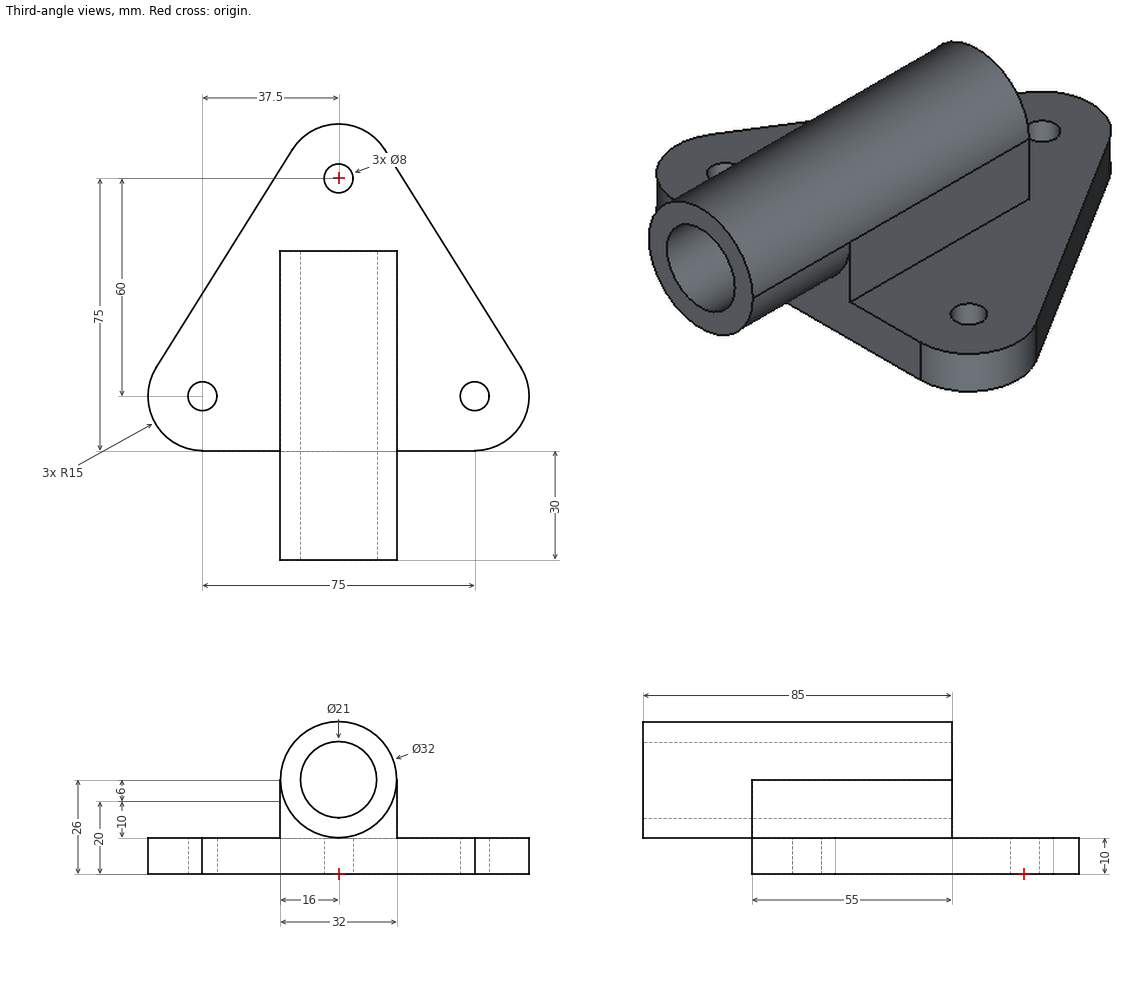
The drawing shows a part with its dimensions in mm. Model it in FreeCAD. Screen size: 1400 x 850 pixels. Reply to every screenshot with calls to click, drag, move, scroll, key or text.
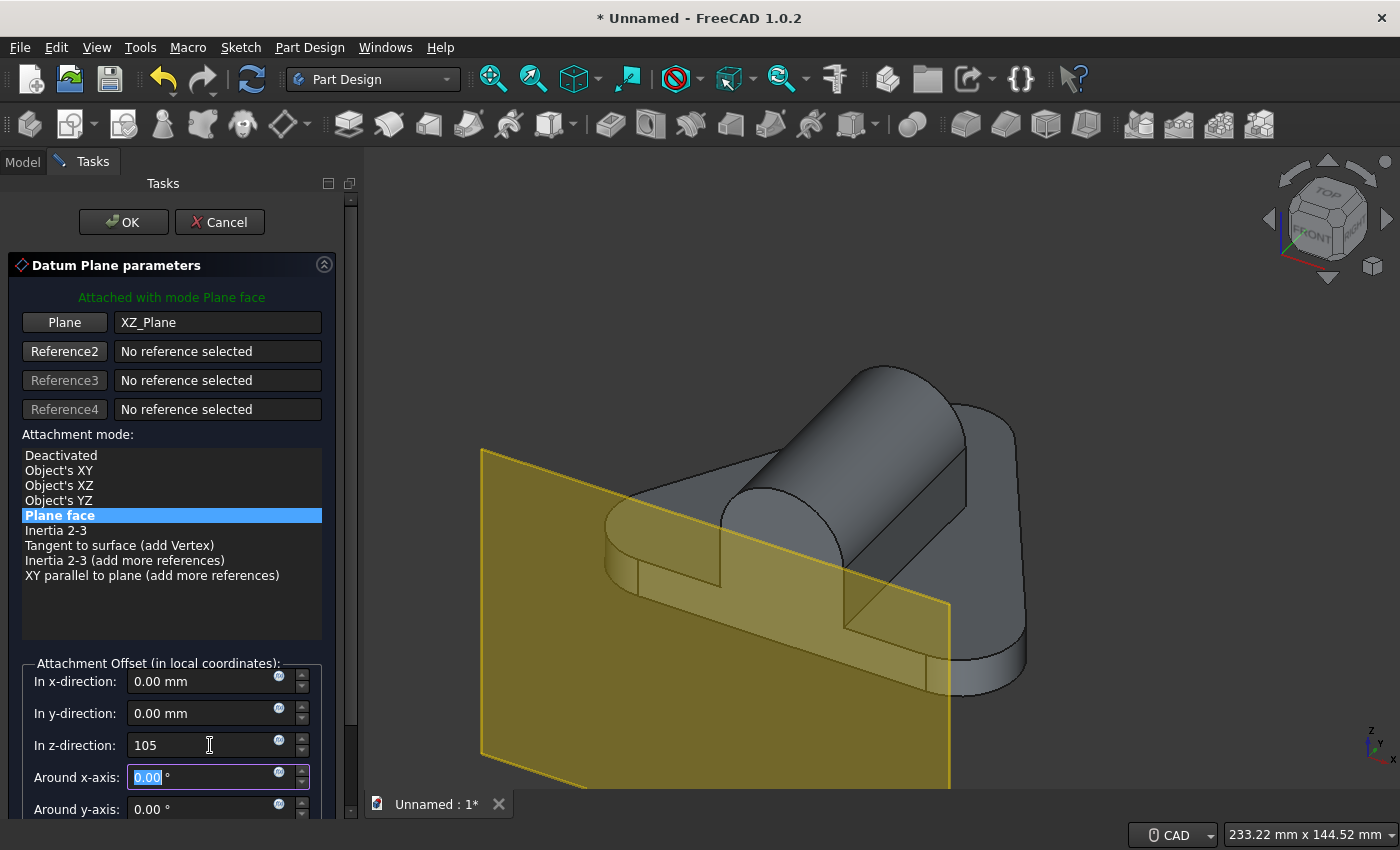
click(124, 222)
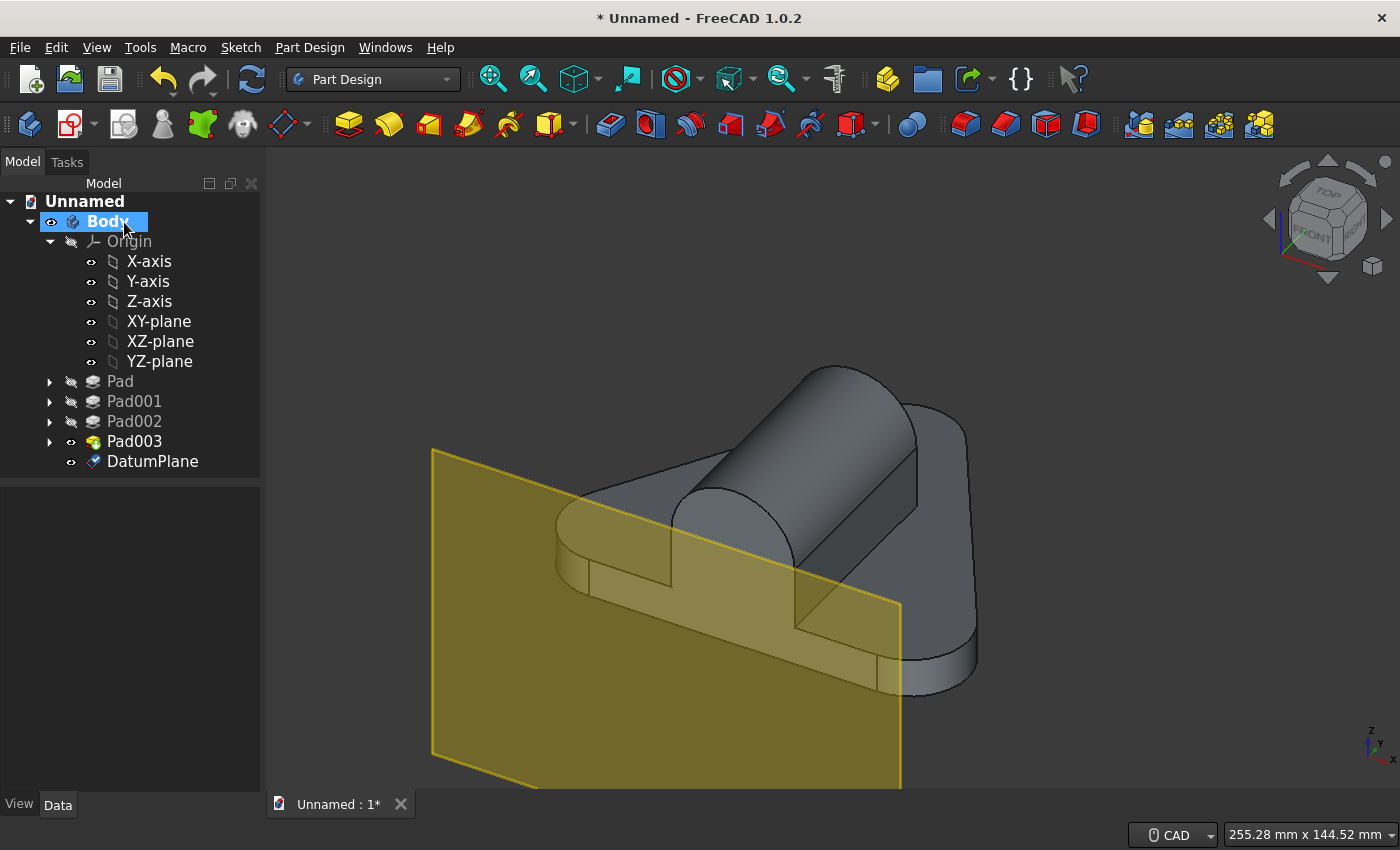
click(116, 462)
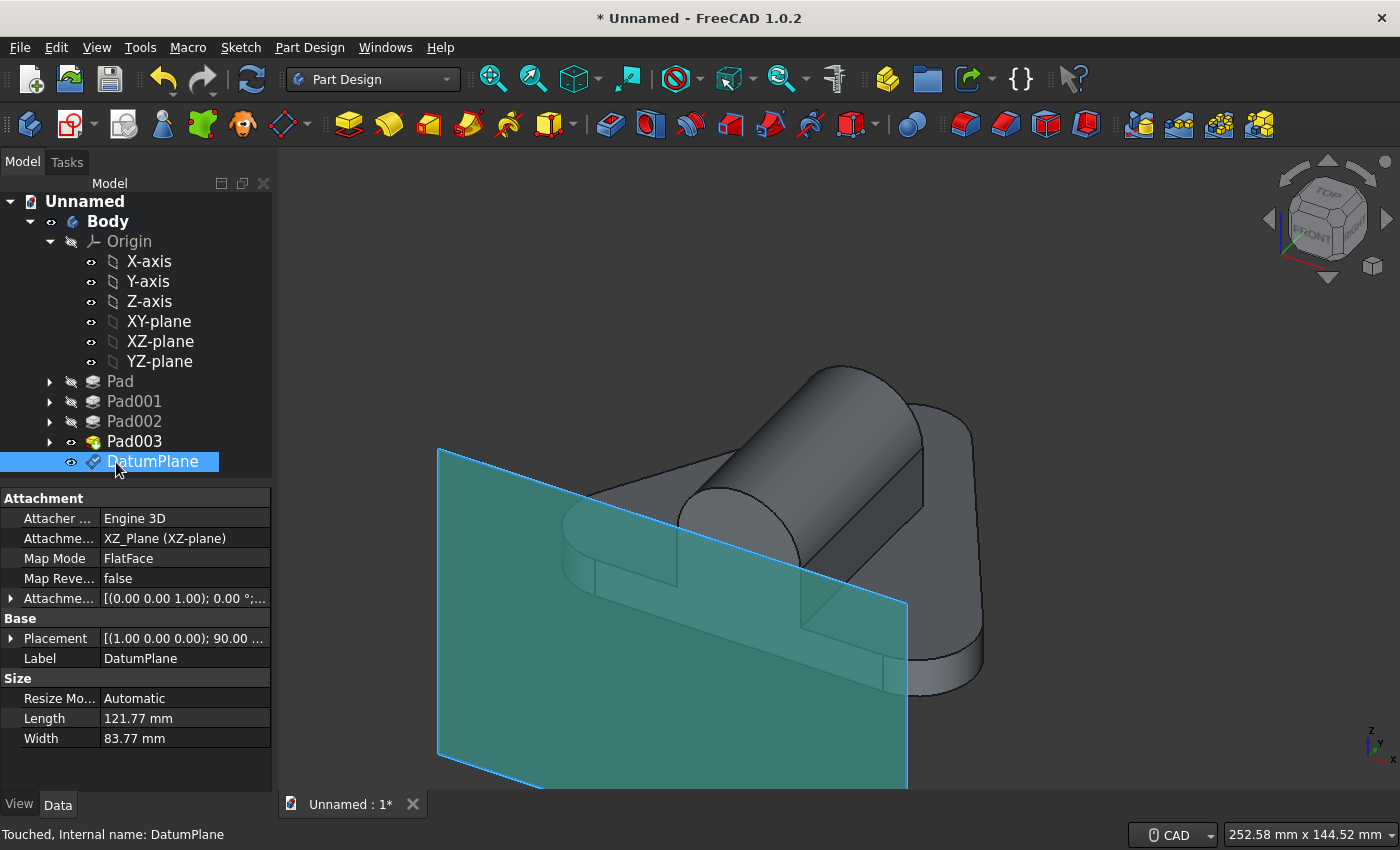
click(70, 124)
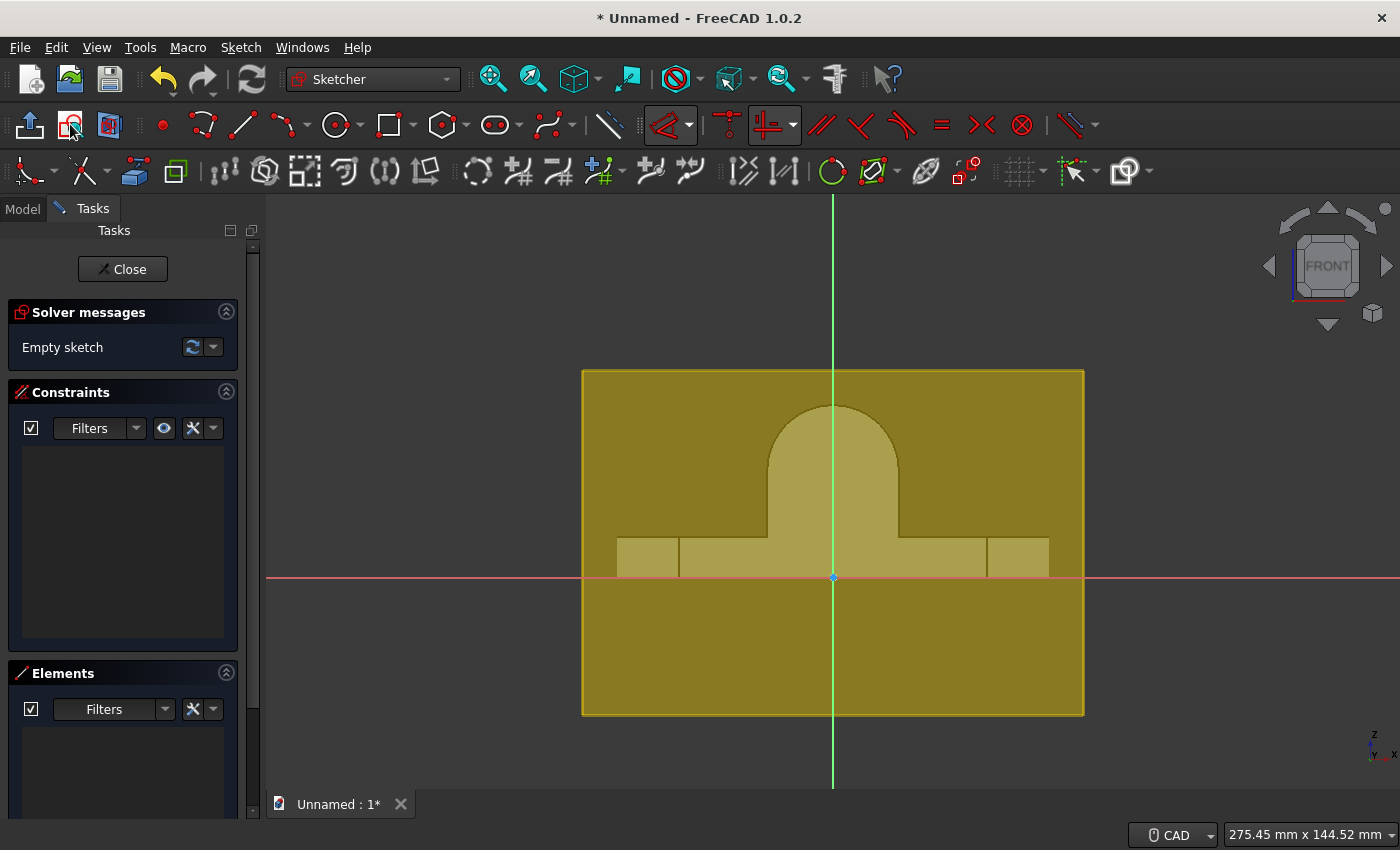
scroll(889, 491, up, 4)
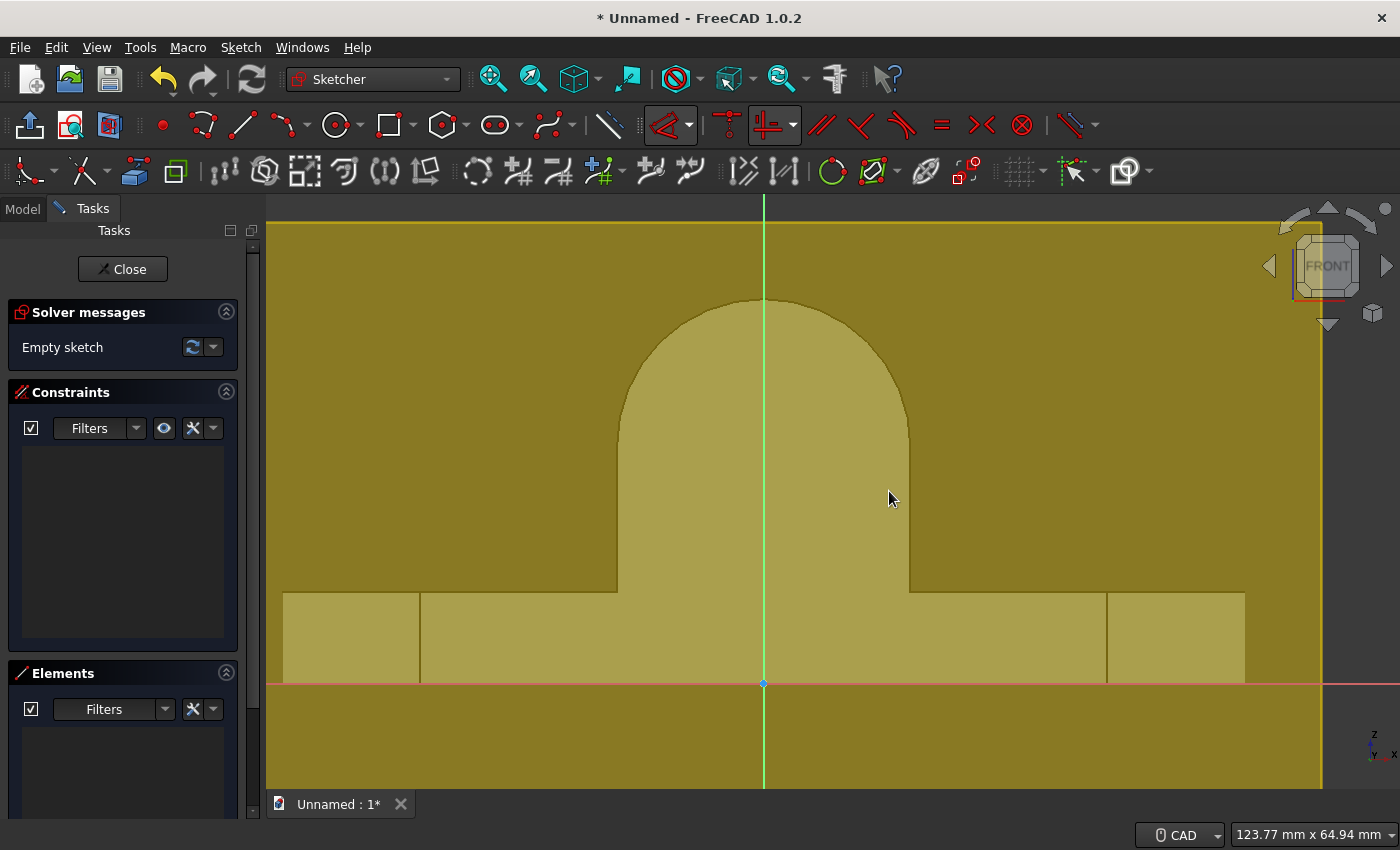
click(336, 126)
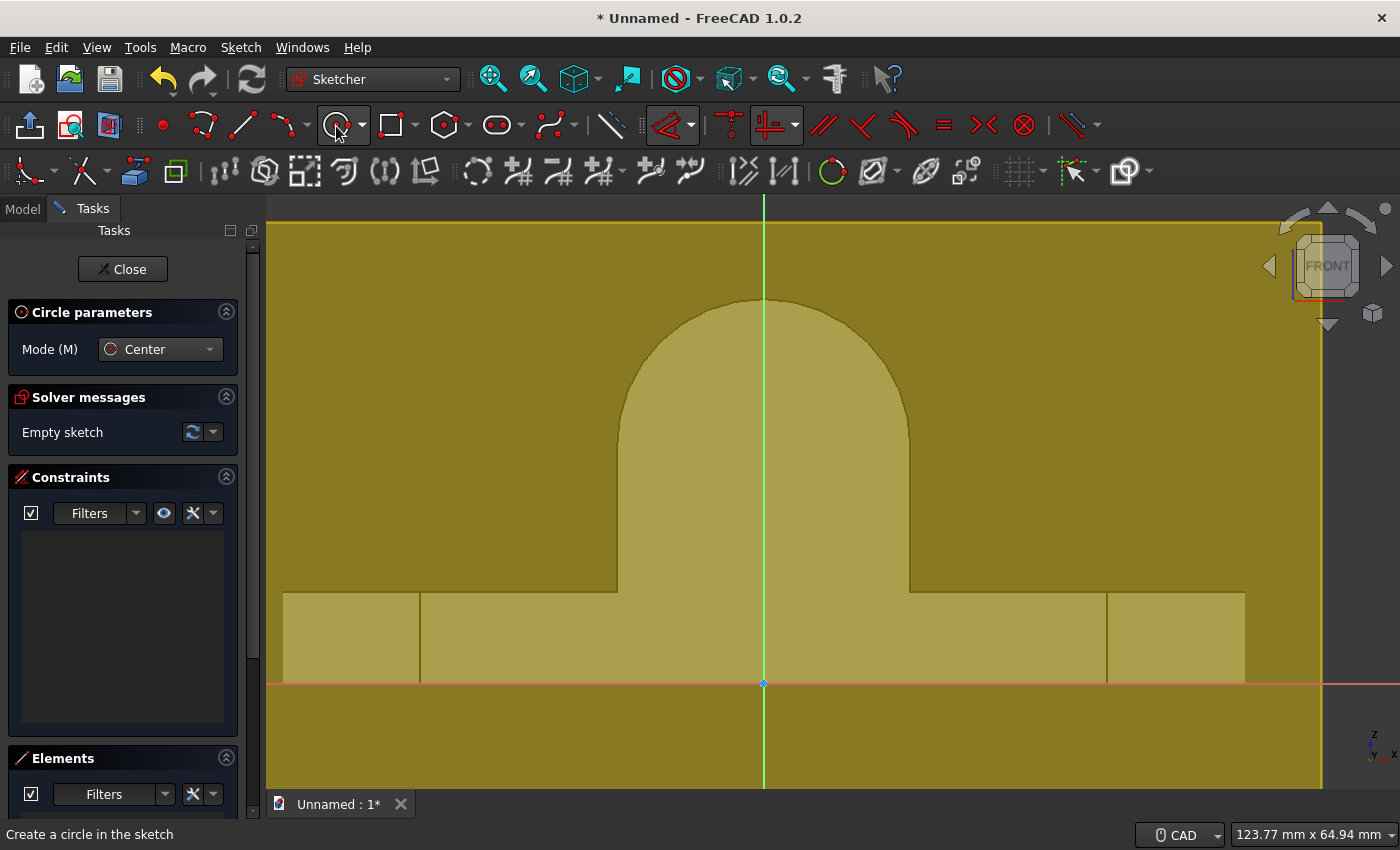
click(764, 446)
click(867, 342)
key(Escape)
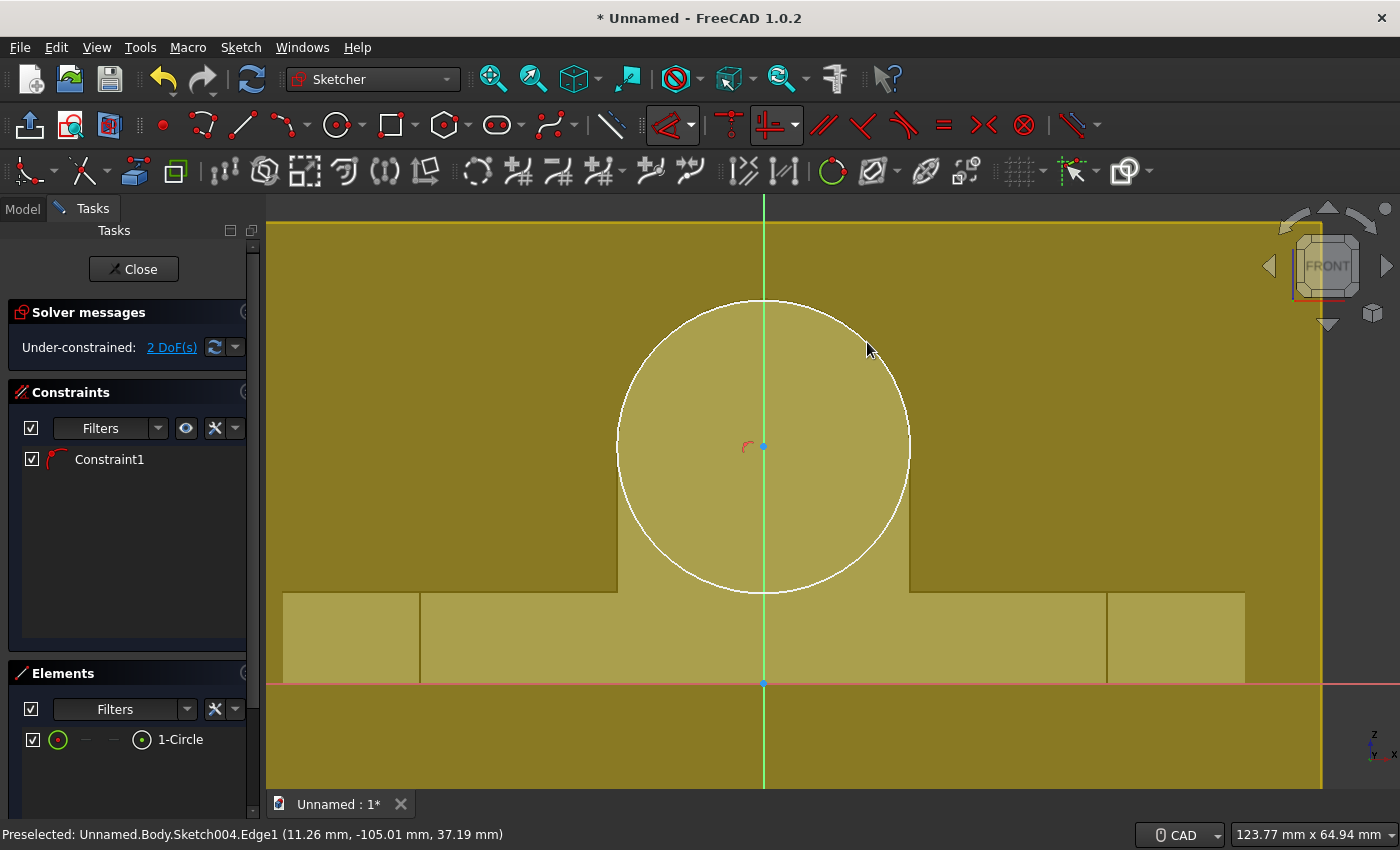
click(867, 343)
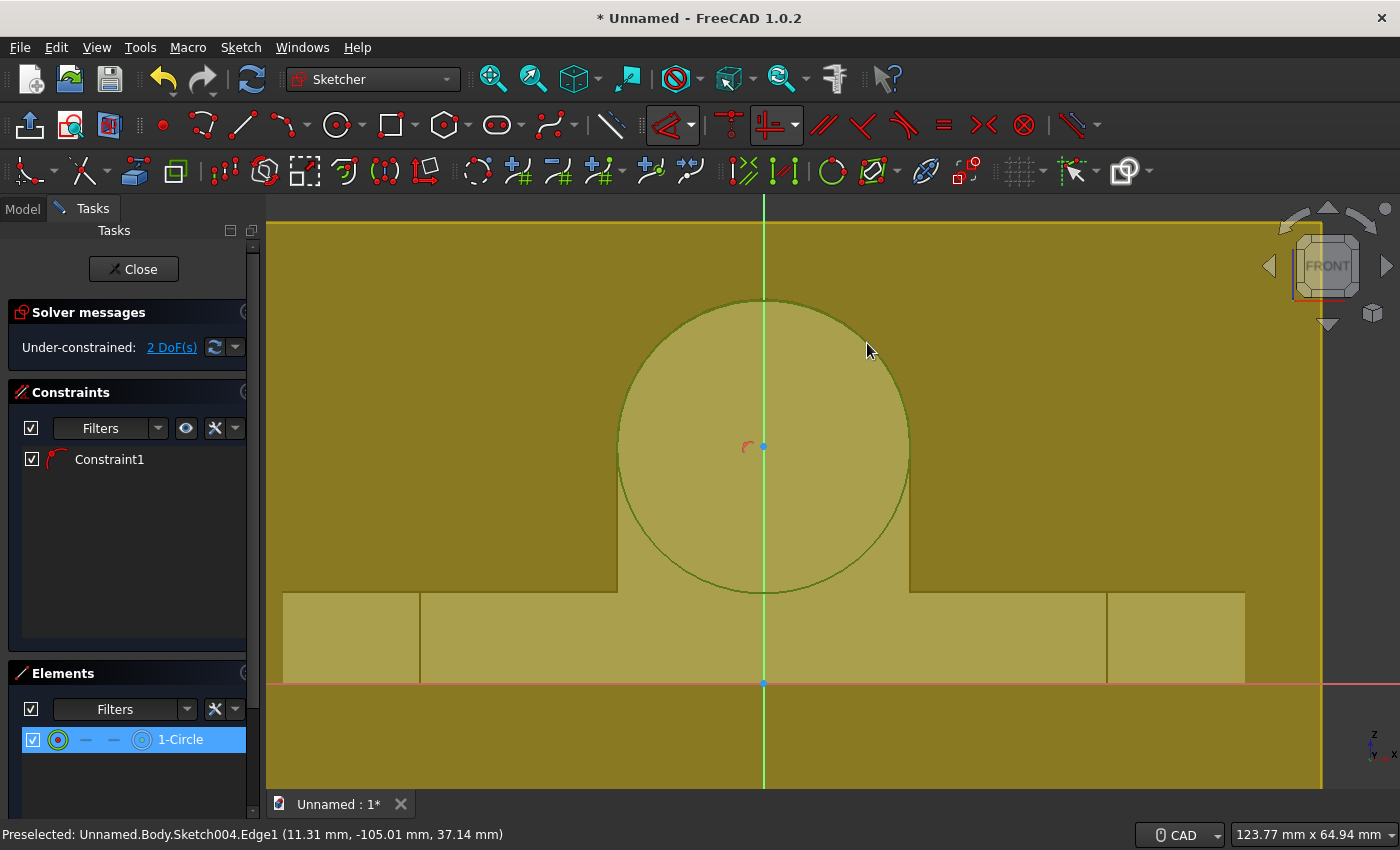
click(694, 126)